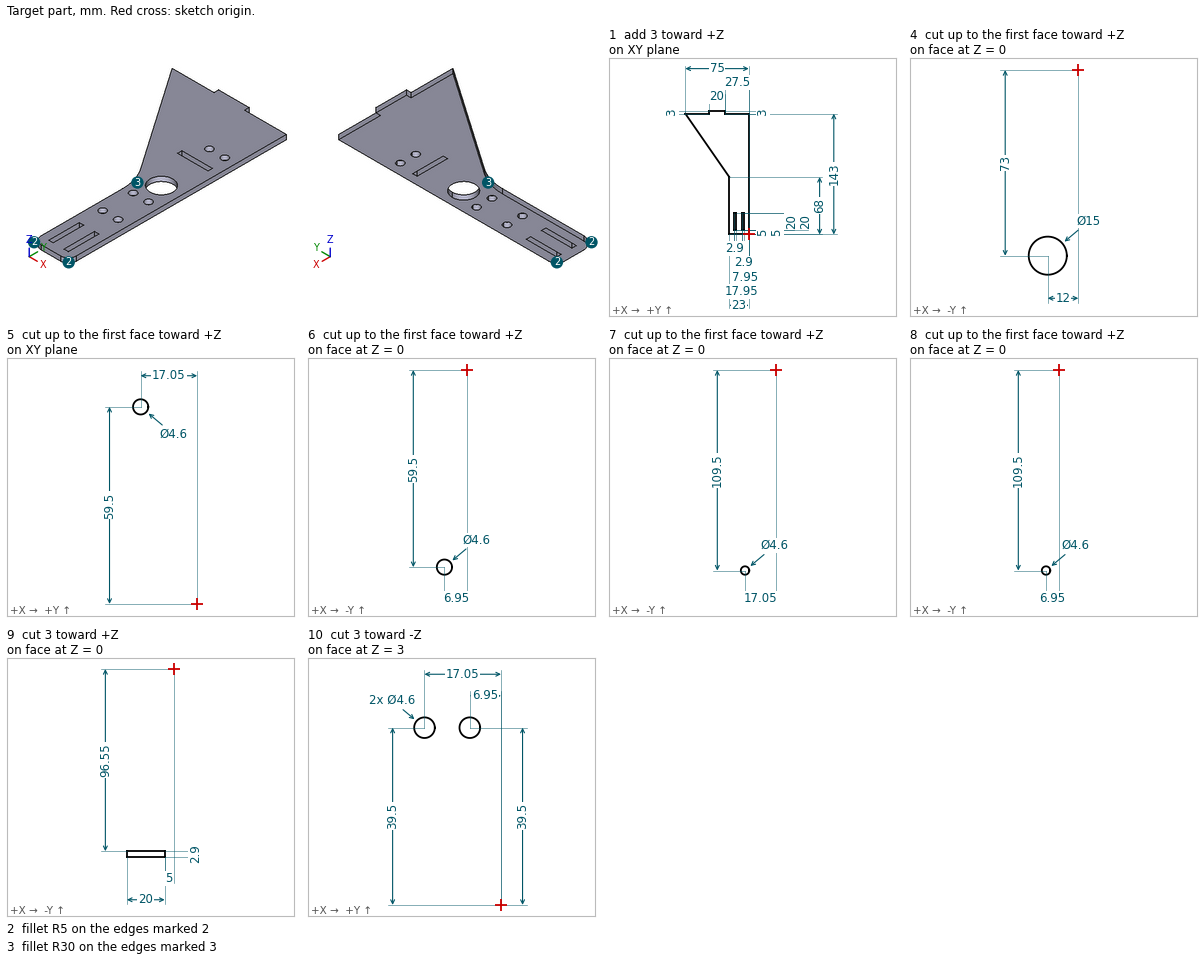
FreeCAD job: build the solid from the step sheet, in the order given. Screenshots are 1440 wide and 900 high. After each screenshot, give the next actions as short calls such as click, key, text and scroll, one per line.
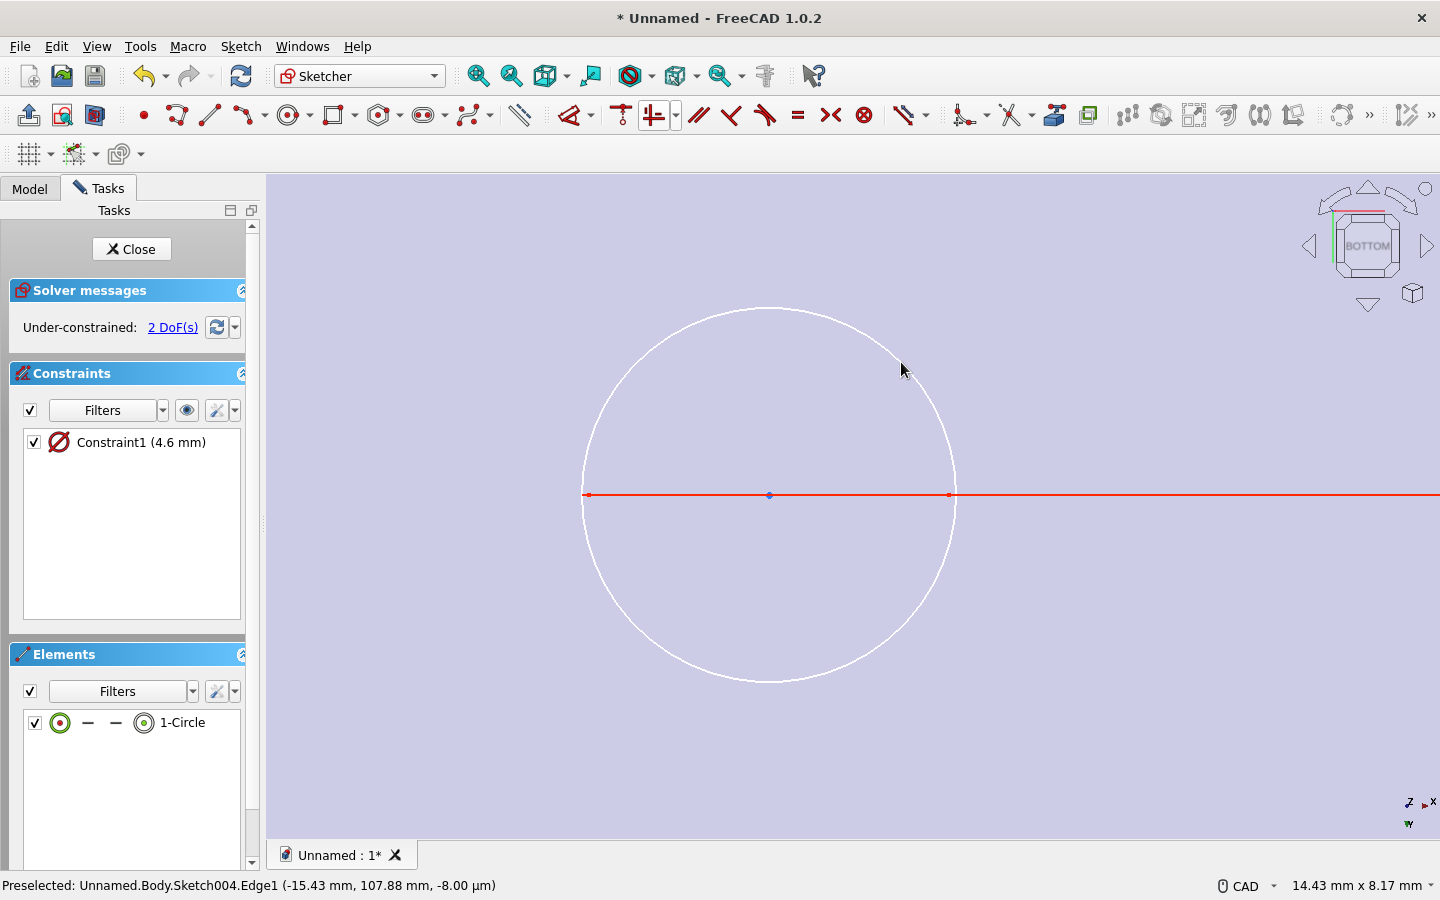
key(d)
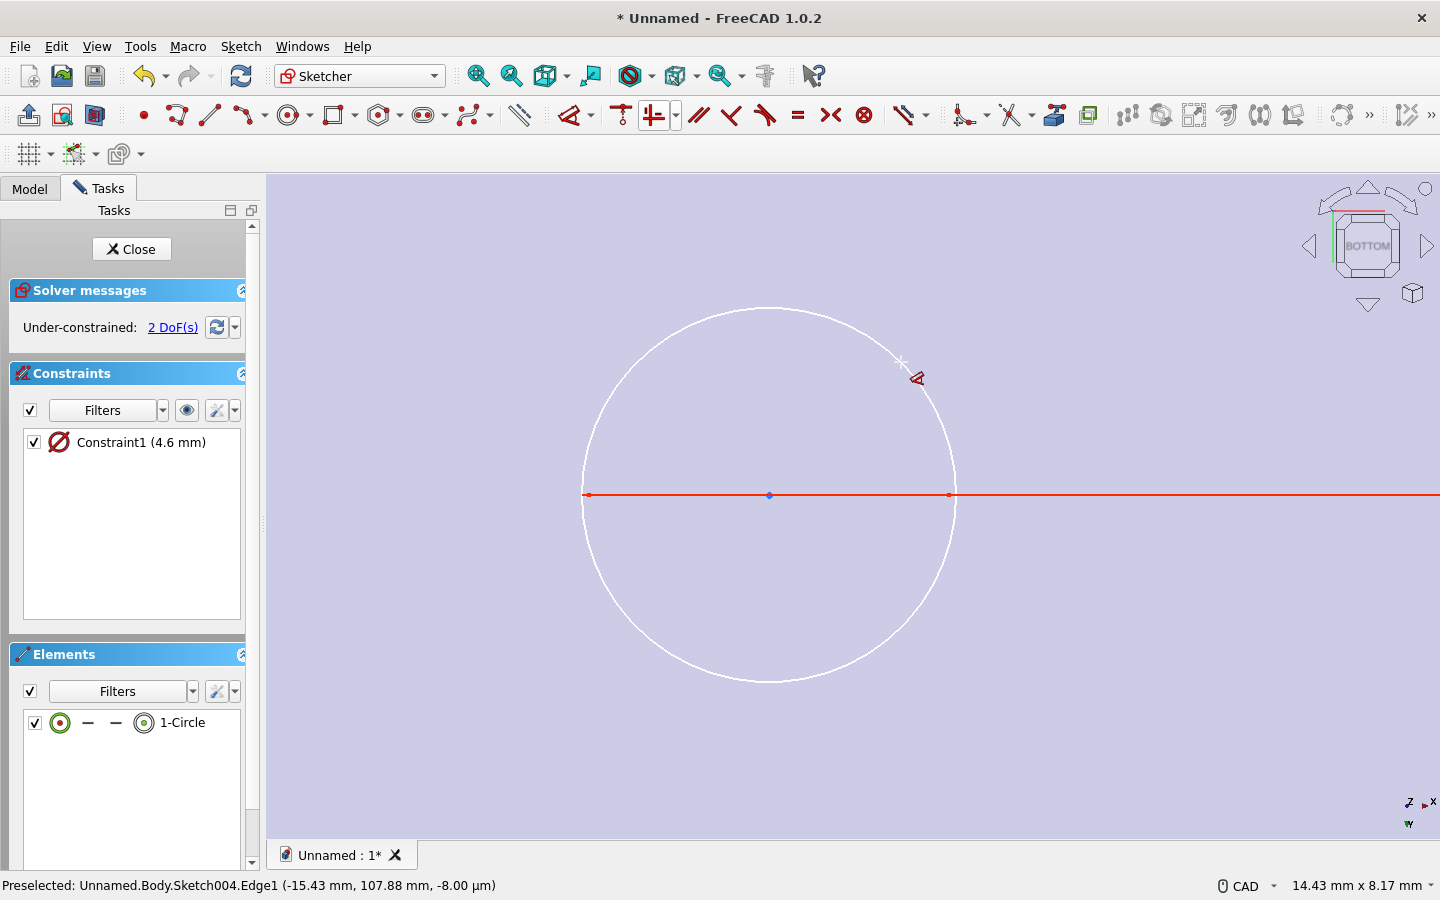
click(769, 495)
click(1022, 529)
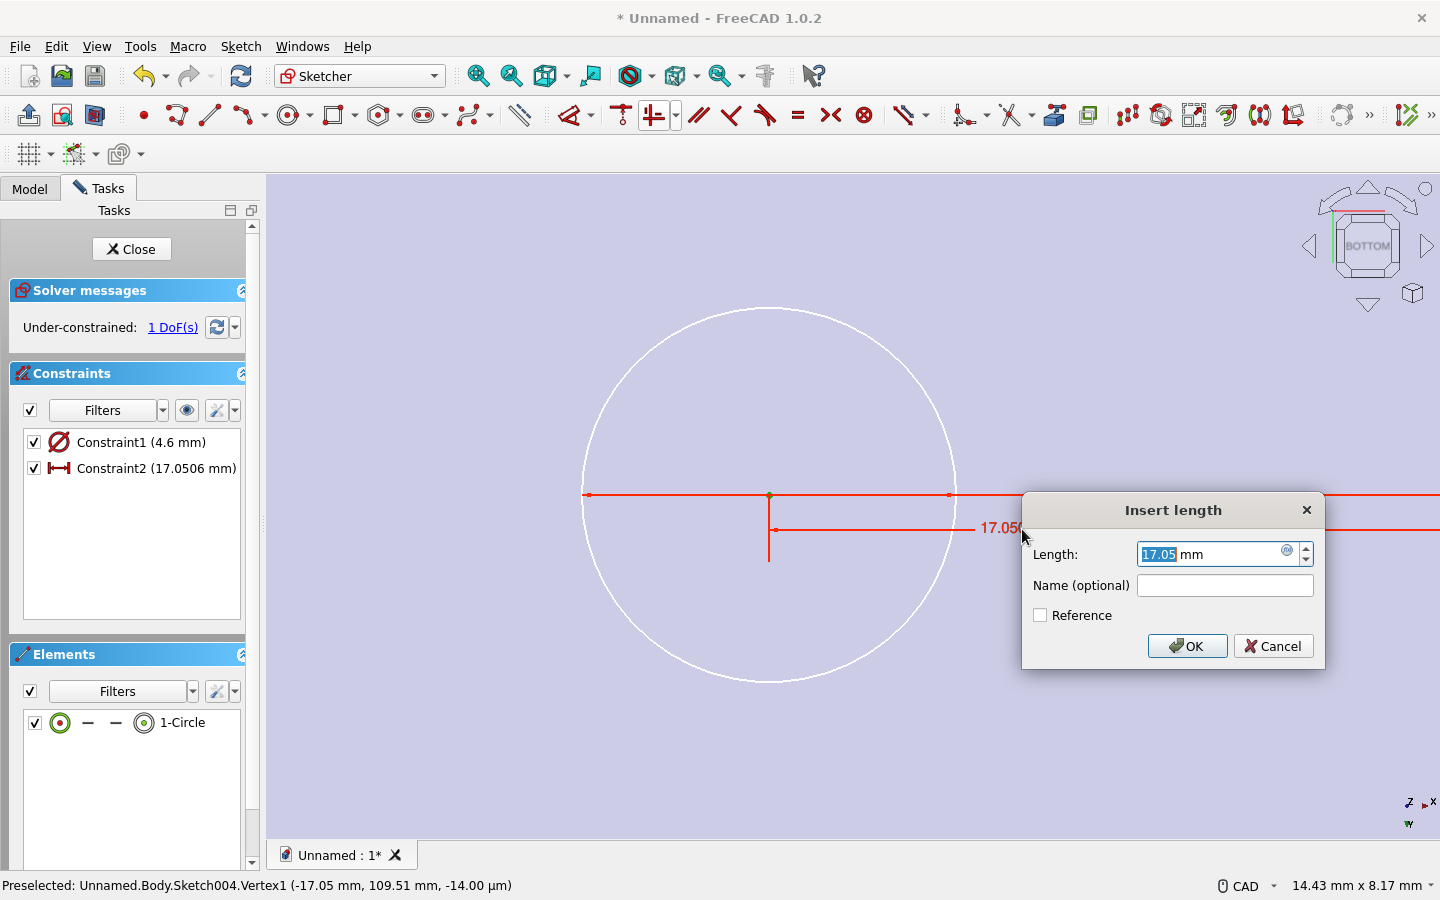
text(17.05)
key(Return)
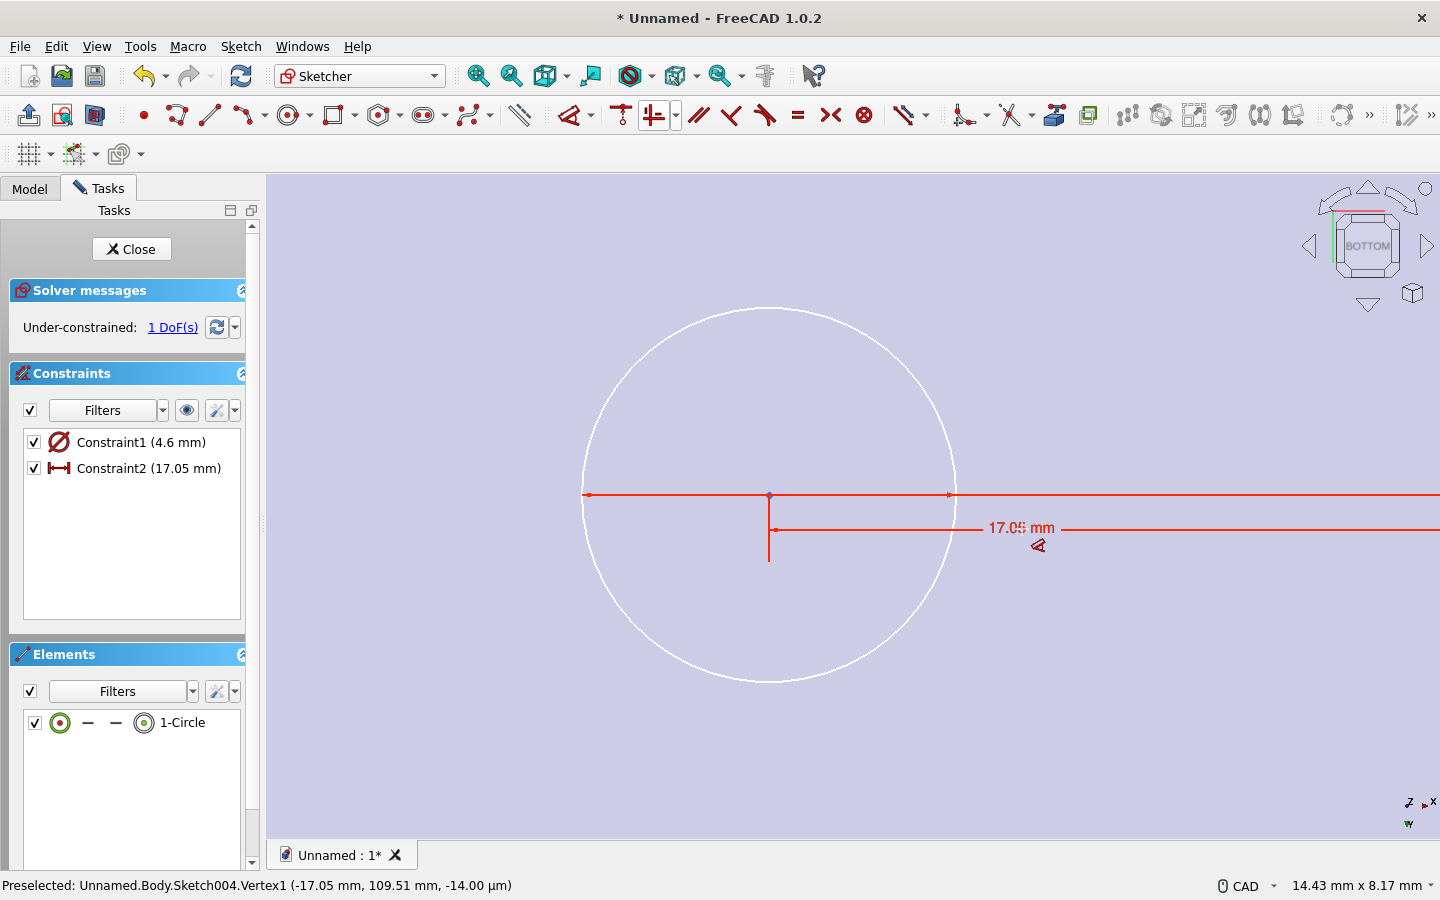
click(769, 495)
click(735, 349)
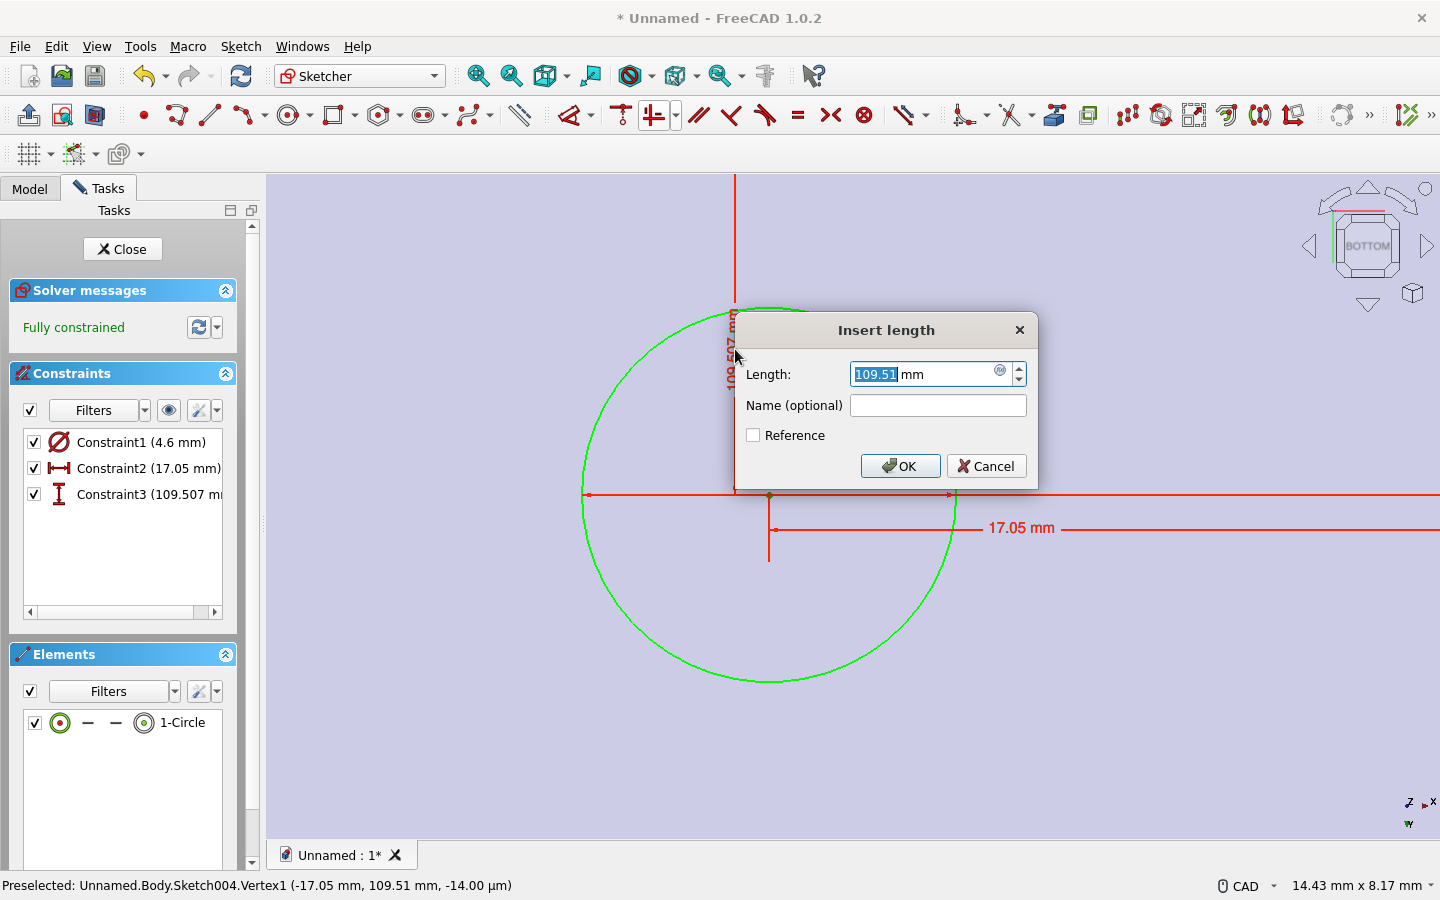
text(109.5)
key(Return)
key(Escape)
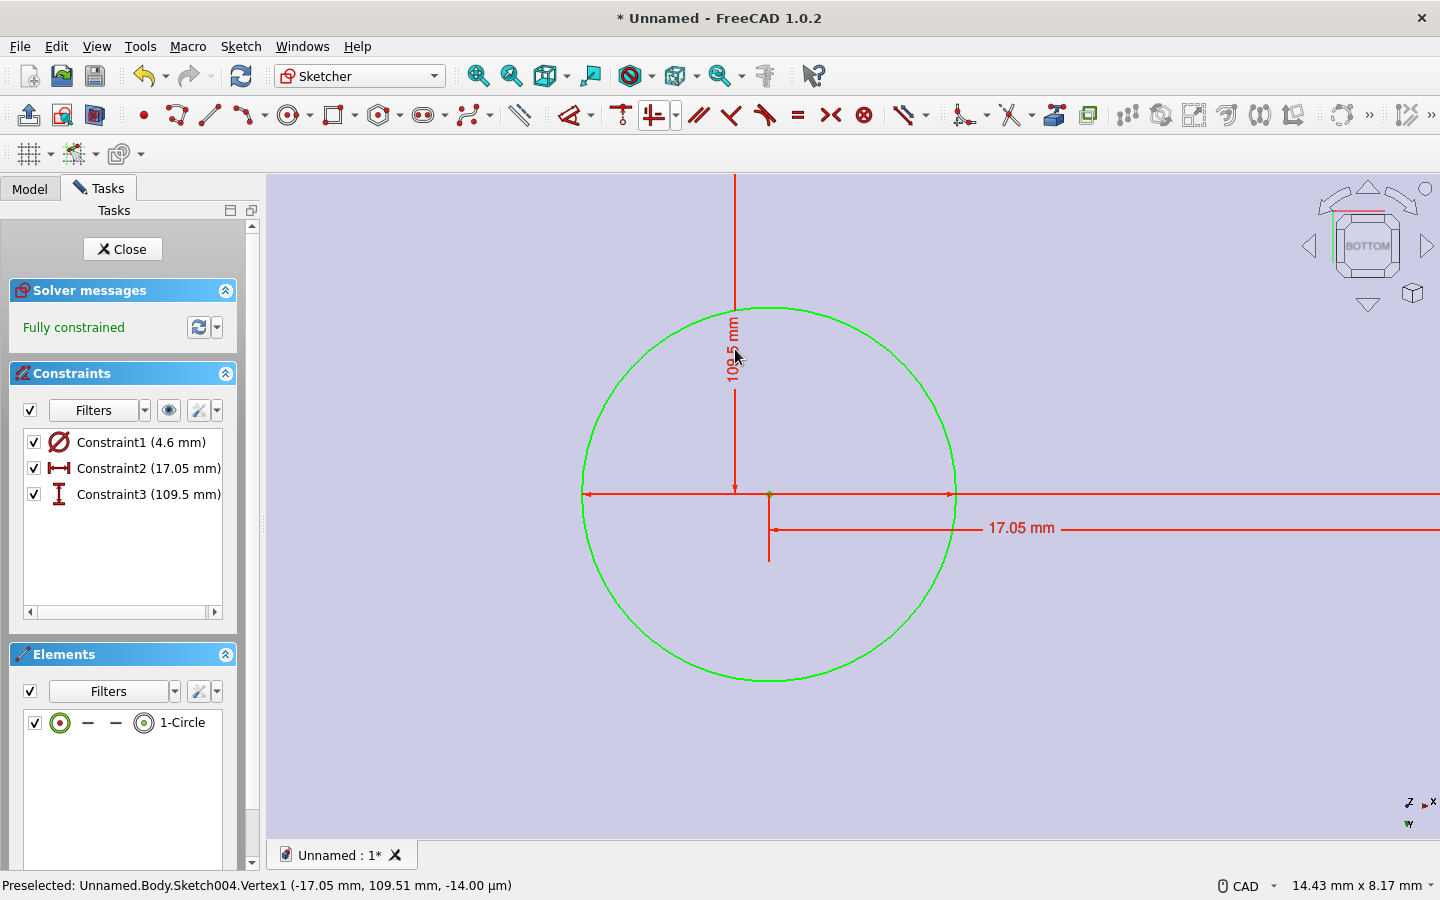
click(123, 249)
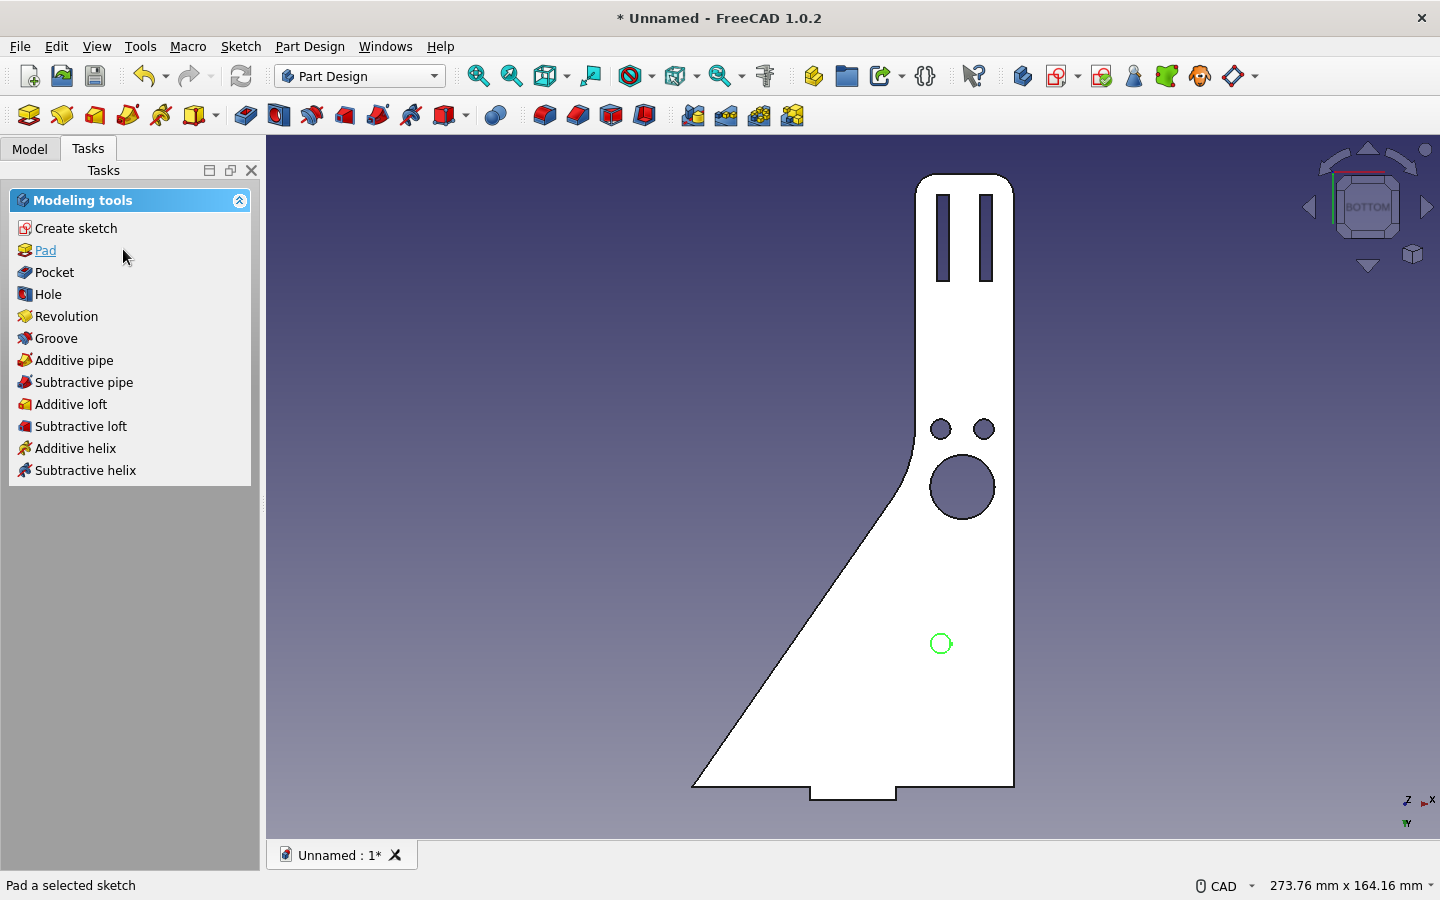
click(246, 116)